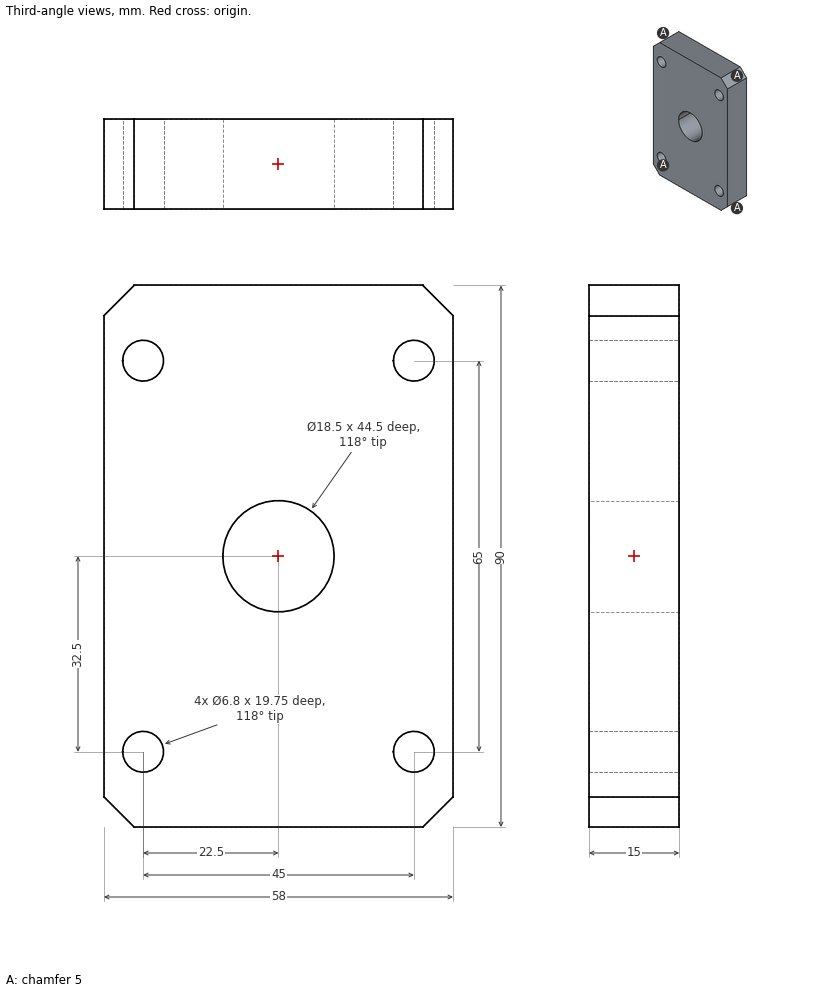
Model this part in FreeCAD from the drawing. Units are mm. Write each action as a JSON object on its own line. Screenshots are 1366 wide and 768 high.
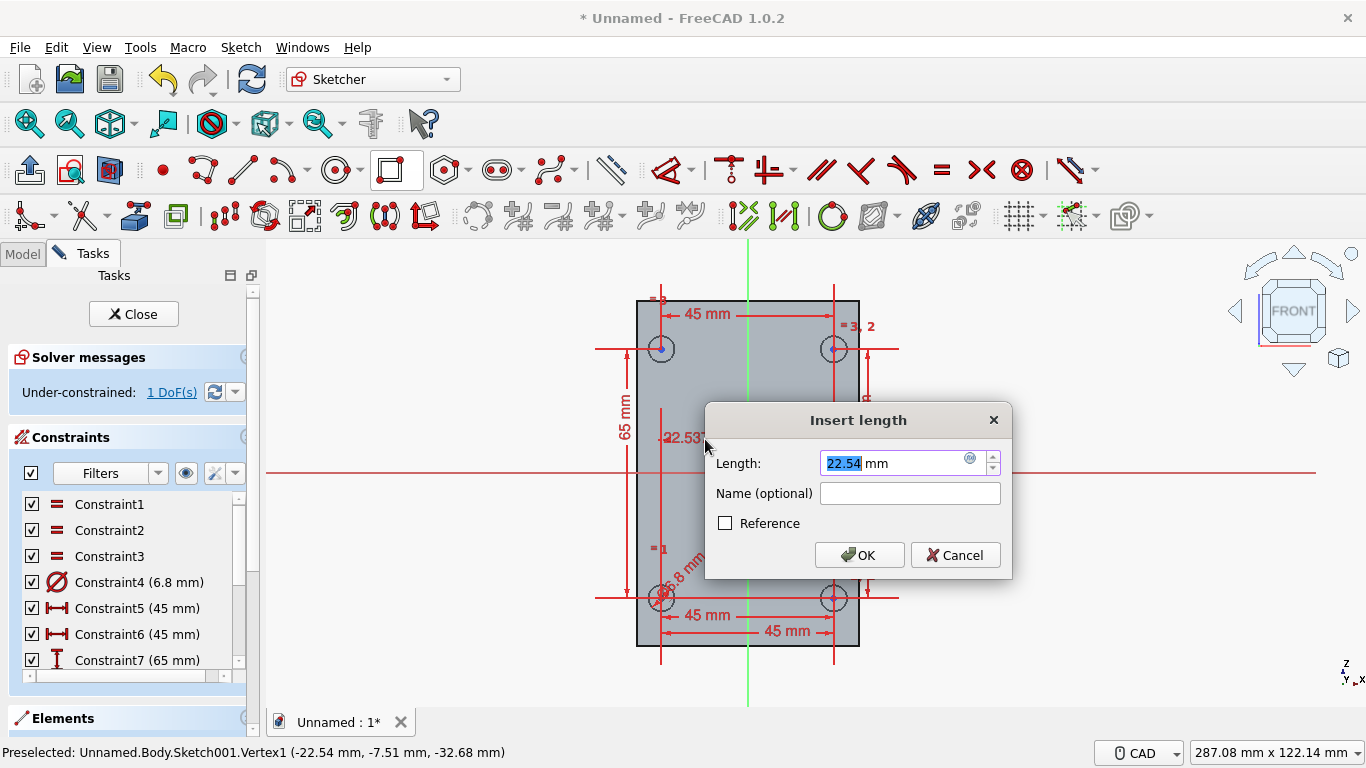
{"action": "type", "text": "22.5"}
{"action": "key", "text": "Return"}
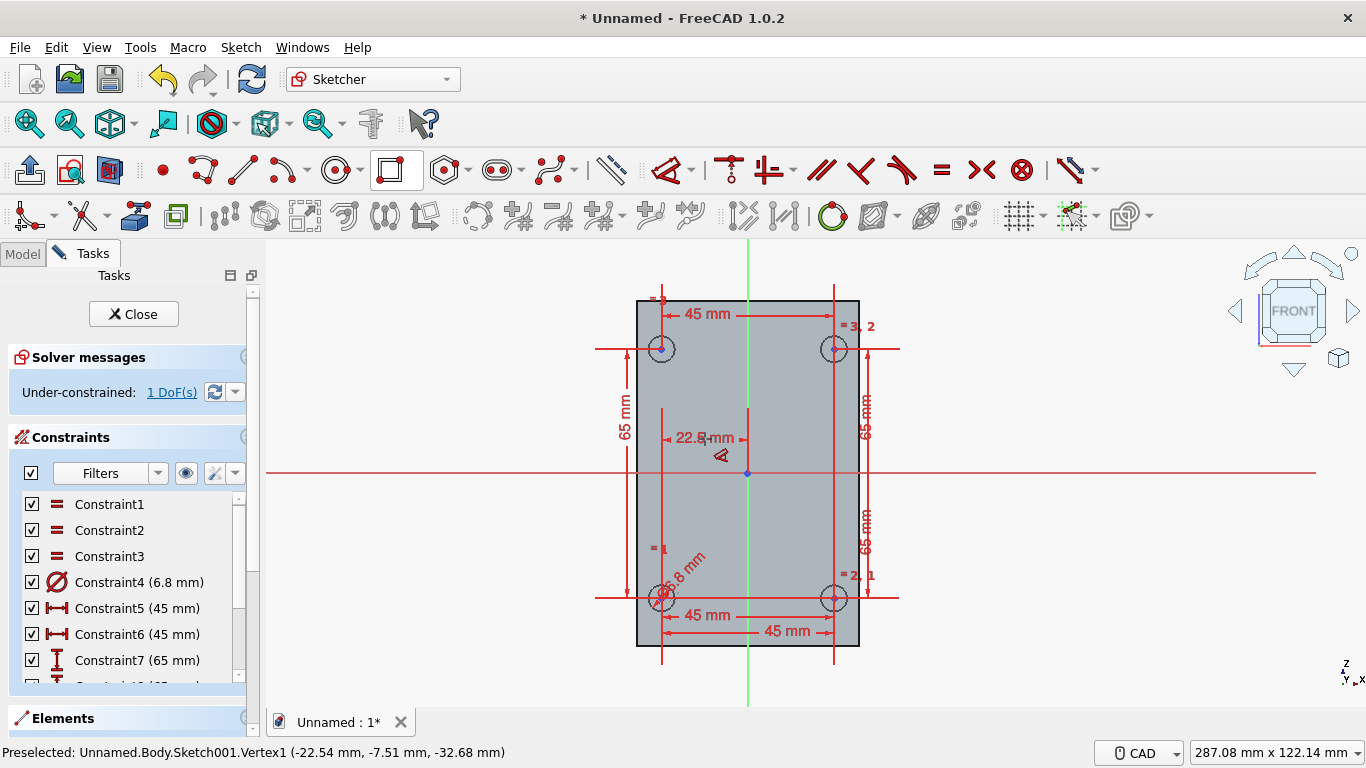
{"action": "left_click", "coordinate": [662, 598]}
{"action": "left_click", "coordinate": [628, 536]}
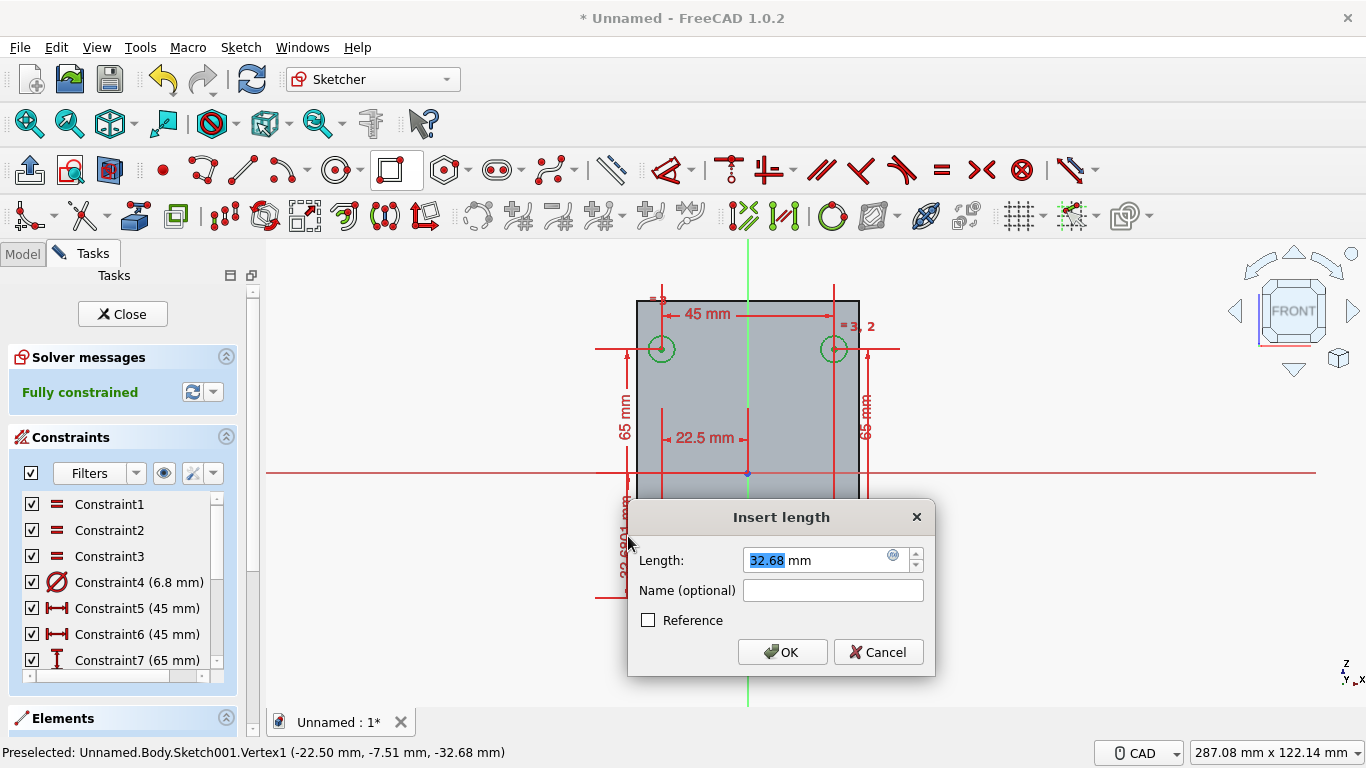
{"action": "type", "text": "32.5"}
{"action": "key", "text": "Return"}
{"action": "key", "text": "Escape"}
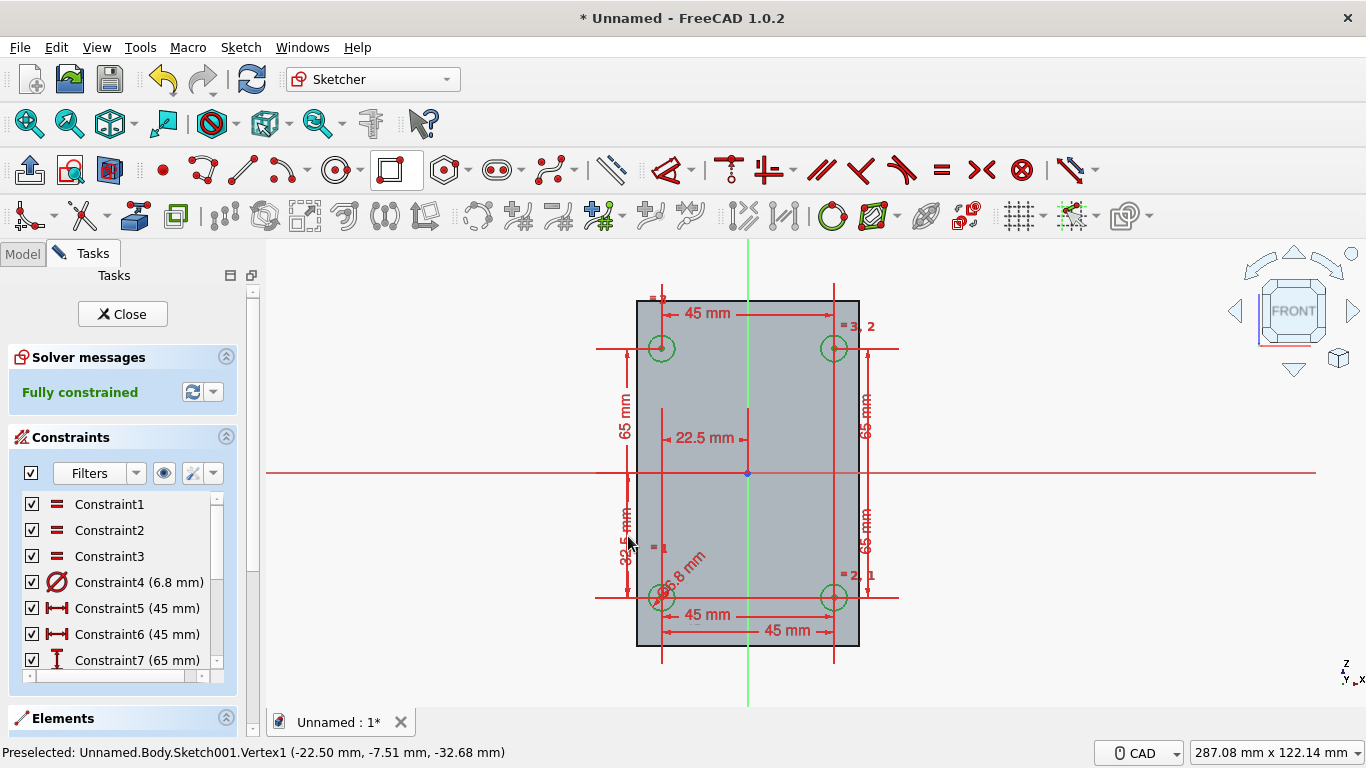
{"action": "left_click", "coordinate": [123, 314]}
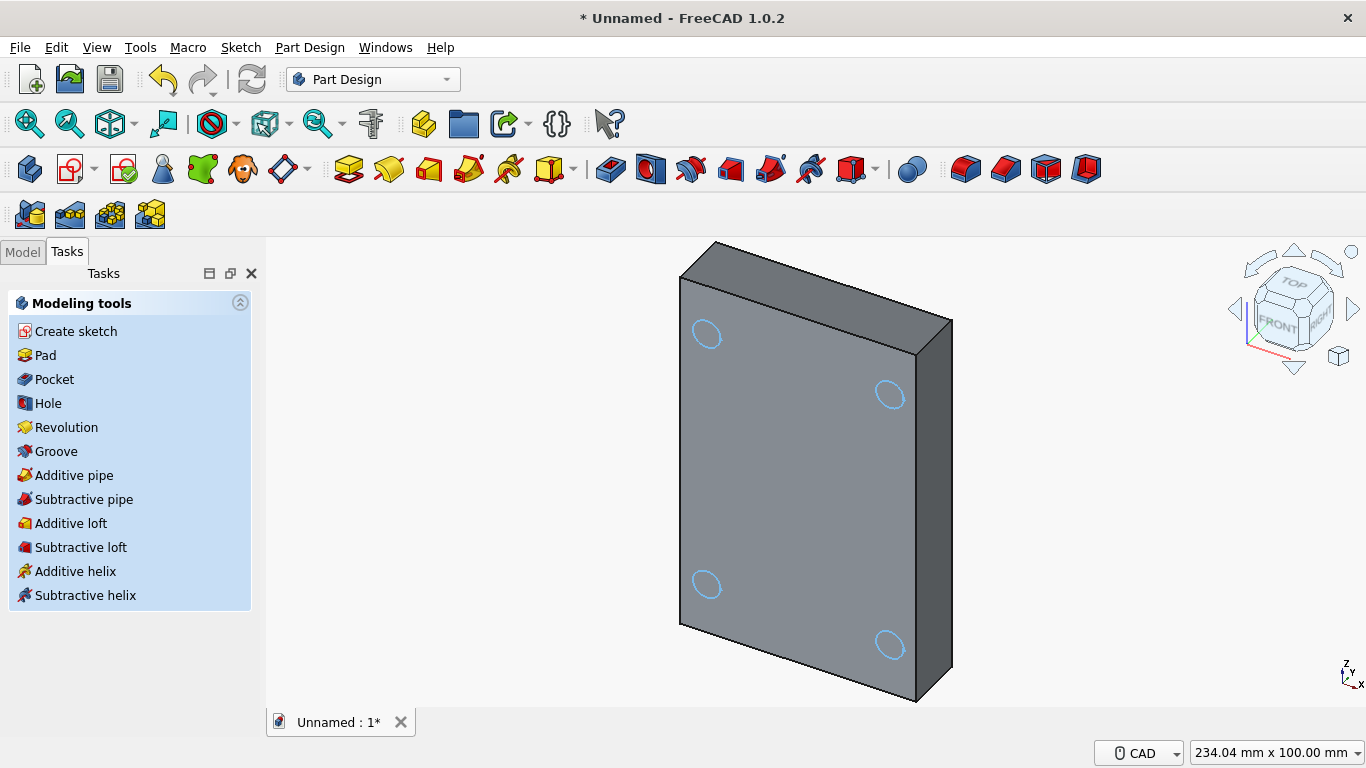
{"action": "left_click", "coordinate": [652, 170]}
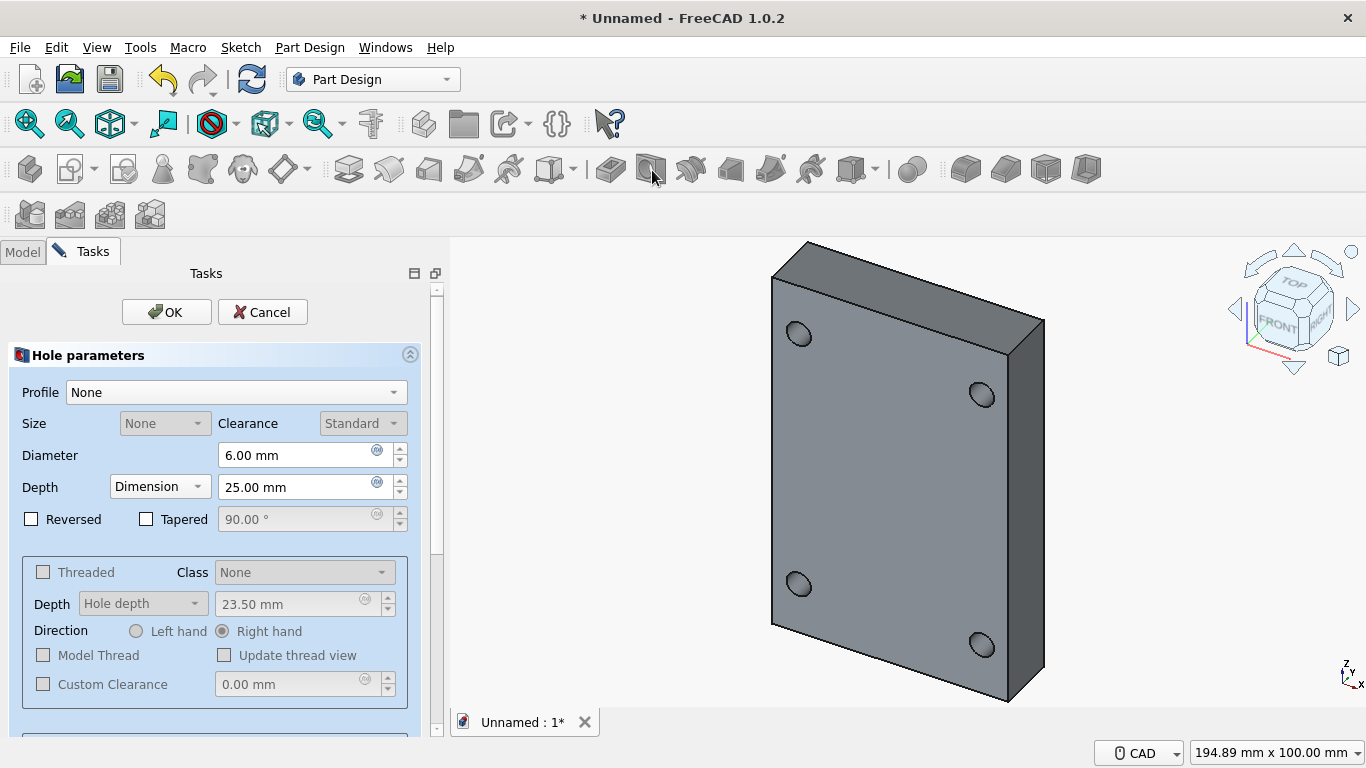
{"action": "triple_click", "coordinate": [305, 455]}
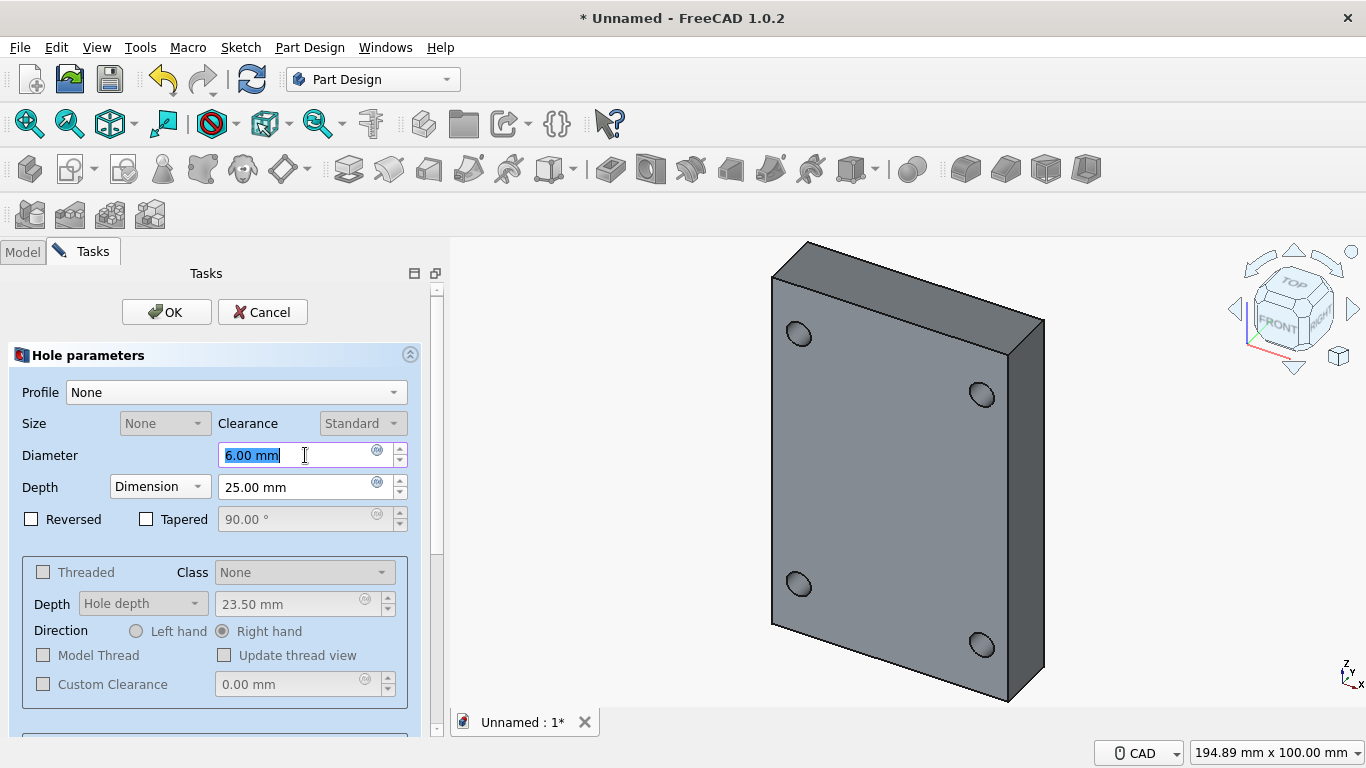
{"action": "type", "text": "6.8"}
{"action": "key", "text": "Tab"}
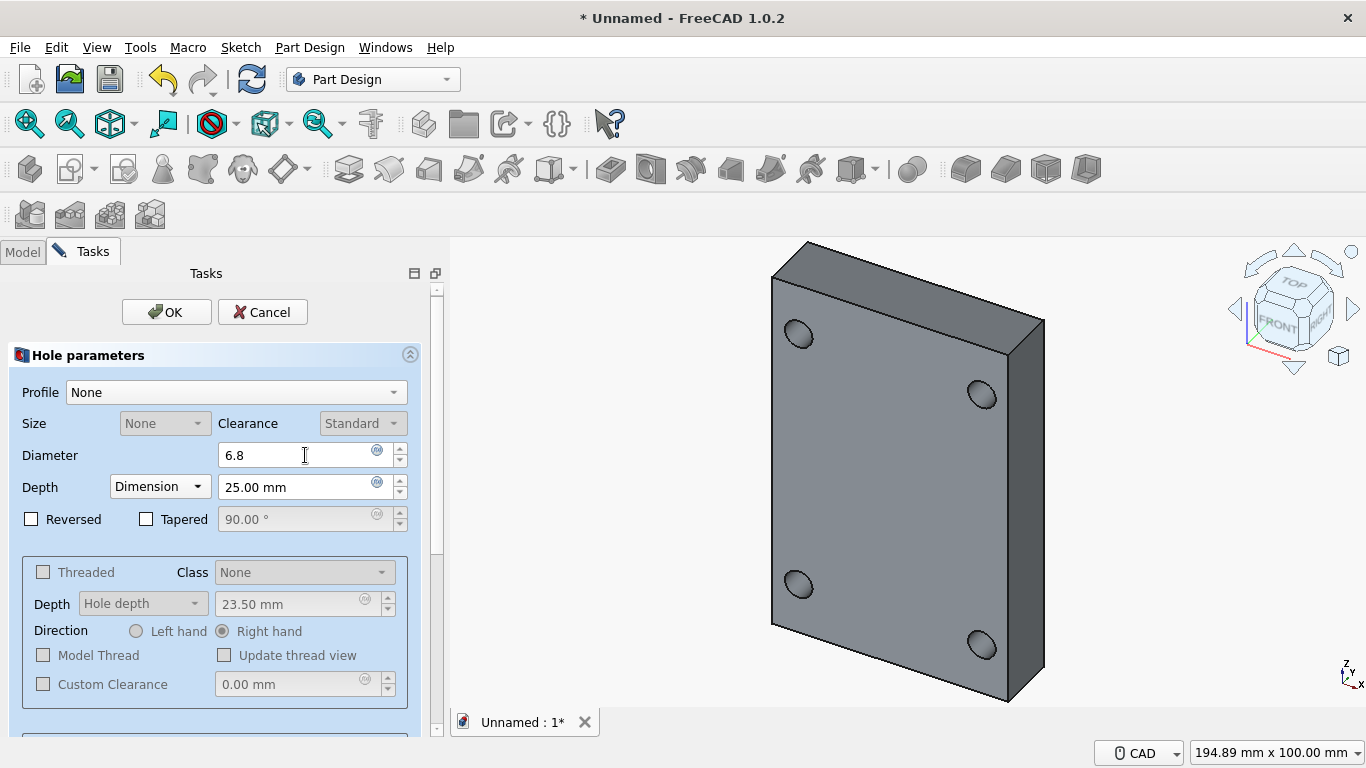
{"action": "triple_click", "coordinate": [305, 487]}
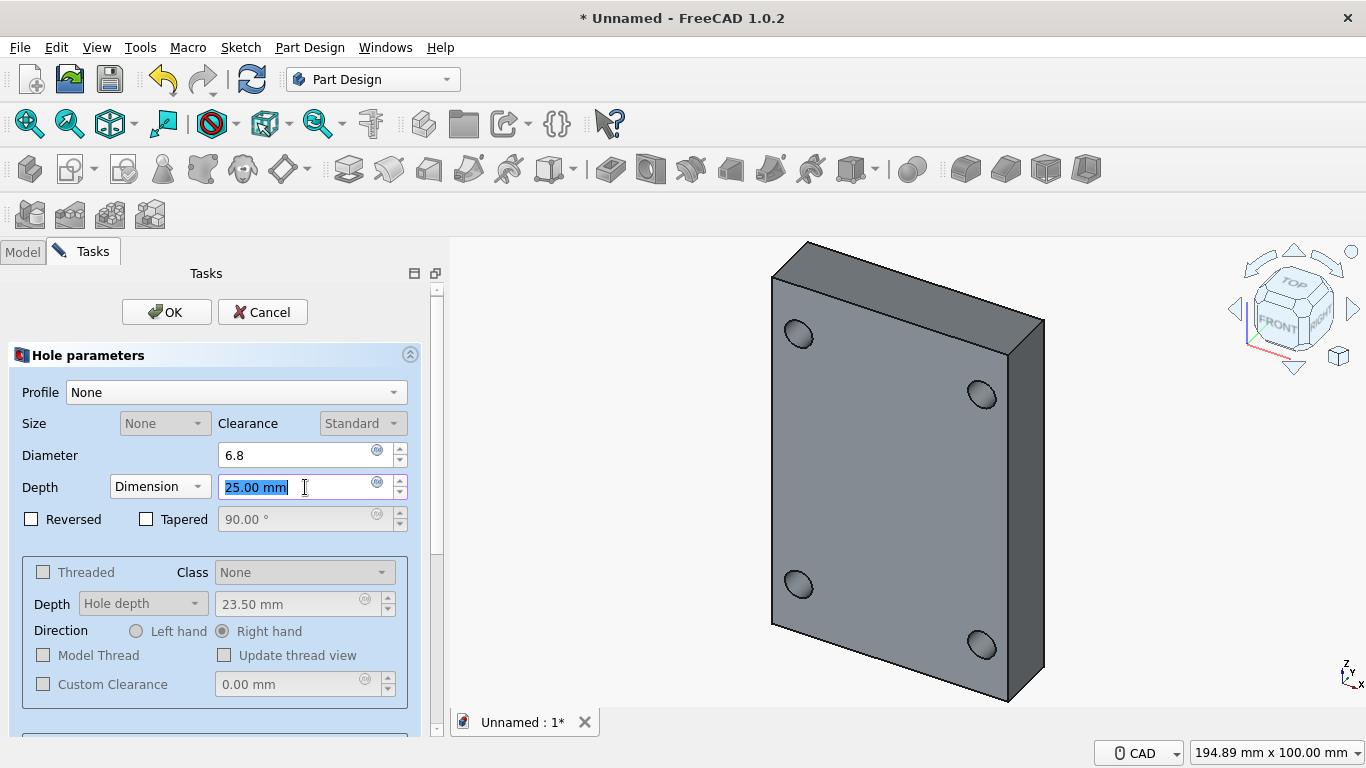
{"action": "type", "text": "19.75"}
{"action": "key", "text": "Tab"}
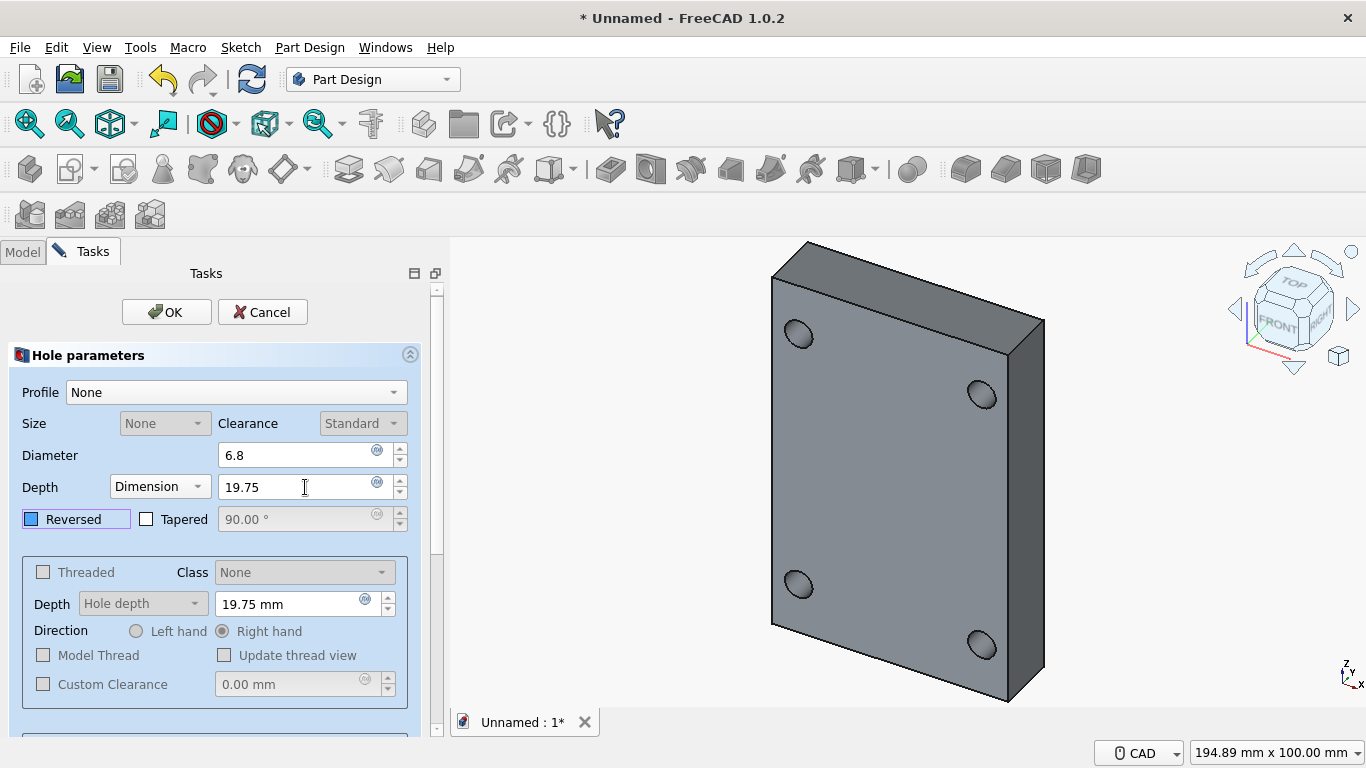
{"action": "left_click", "coordinate": [167, 312]}